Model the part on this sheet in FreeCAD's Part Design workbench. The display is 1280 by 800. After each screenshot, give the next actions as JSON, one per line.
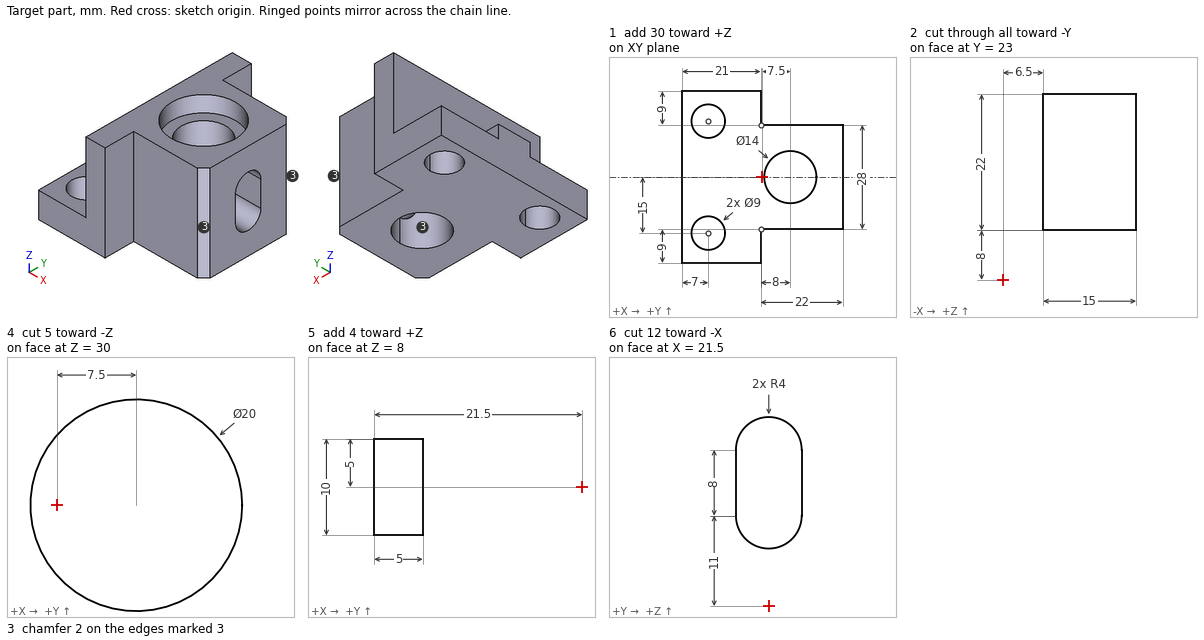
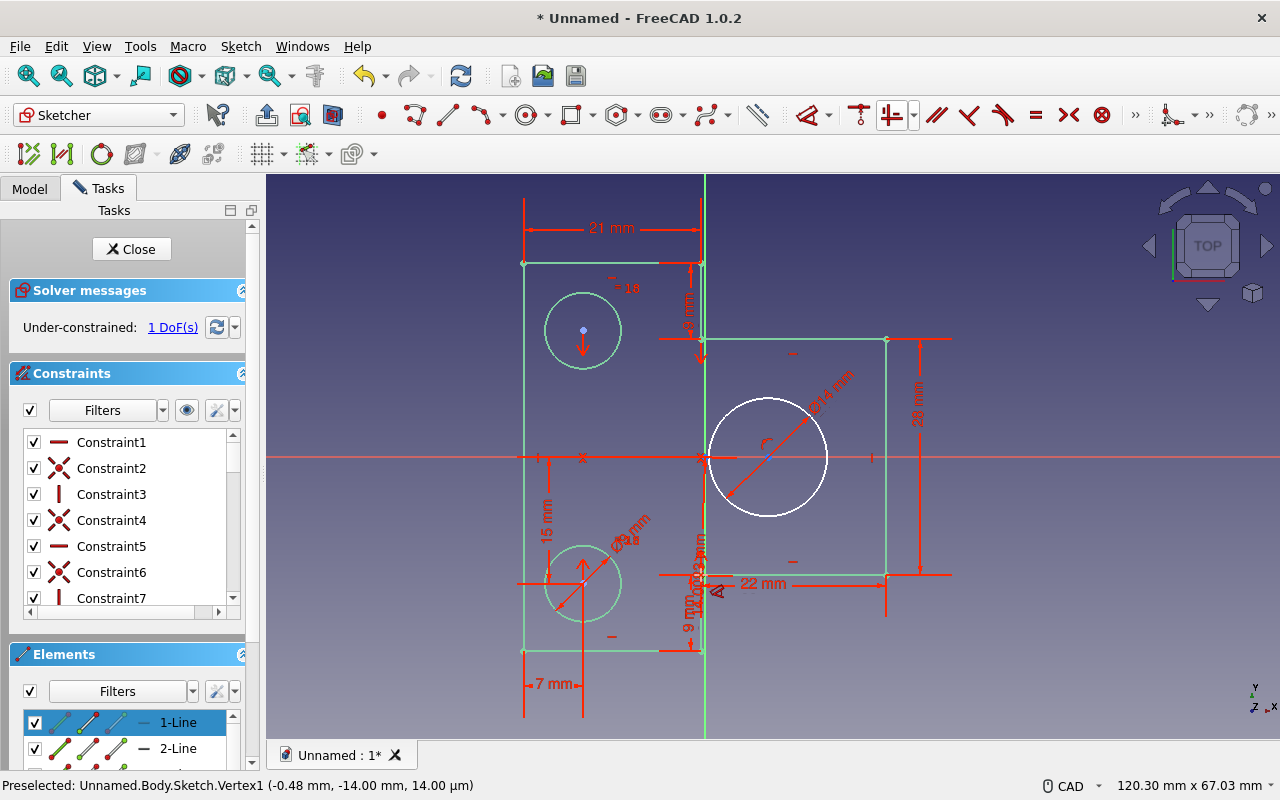
{"action": "left_click", "coordinate": [768, 457]}
{"action": "left_click", "coordinate": [750, 423]}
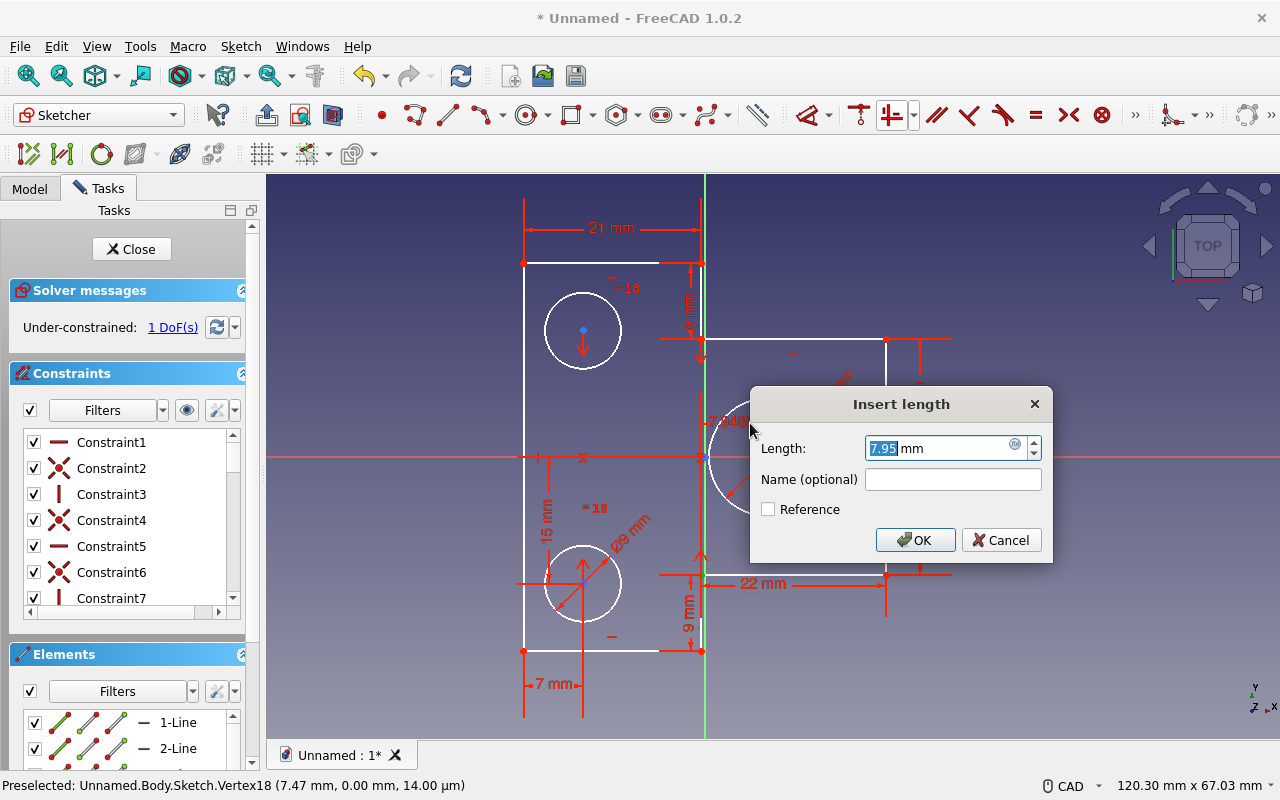
{"action": "type", "text": "8"}
{"action": "key", "text": "Return"}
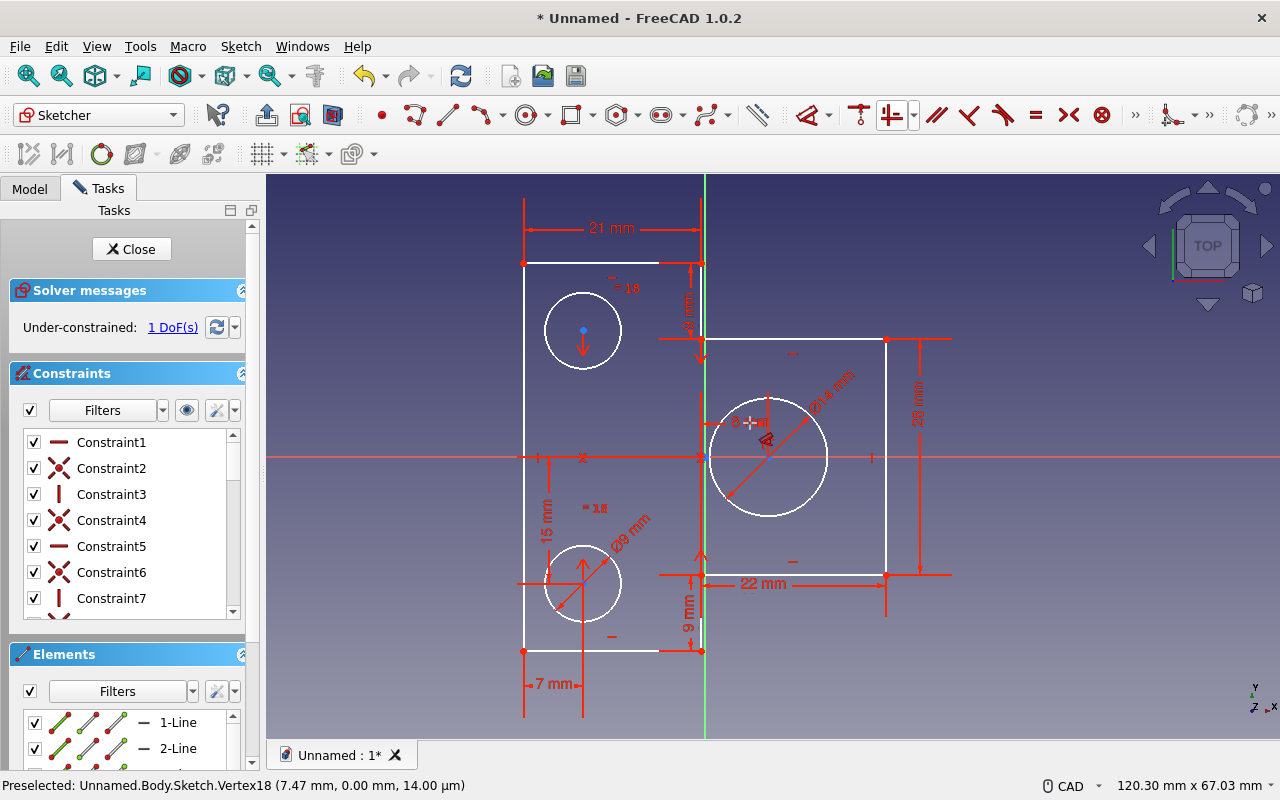
{"action": "left_click", "coordinate": [768, 457]}
{"action": "left_click", "coordinate": [751, 491]}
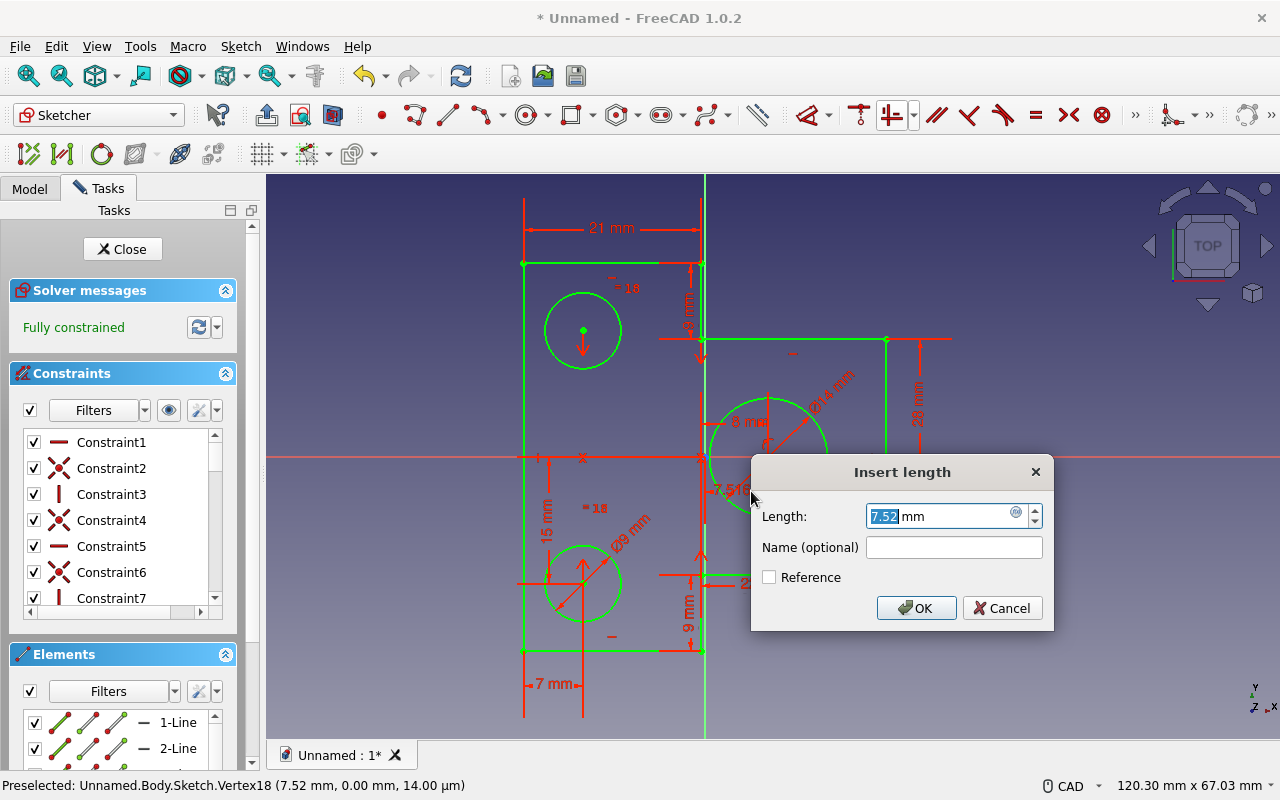
{"action": "type", "text": "7.5"}
{"action": "key", "text": "Return"}
{"action": "key", "text": "Escape"}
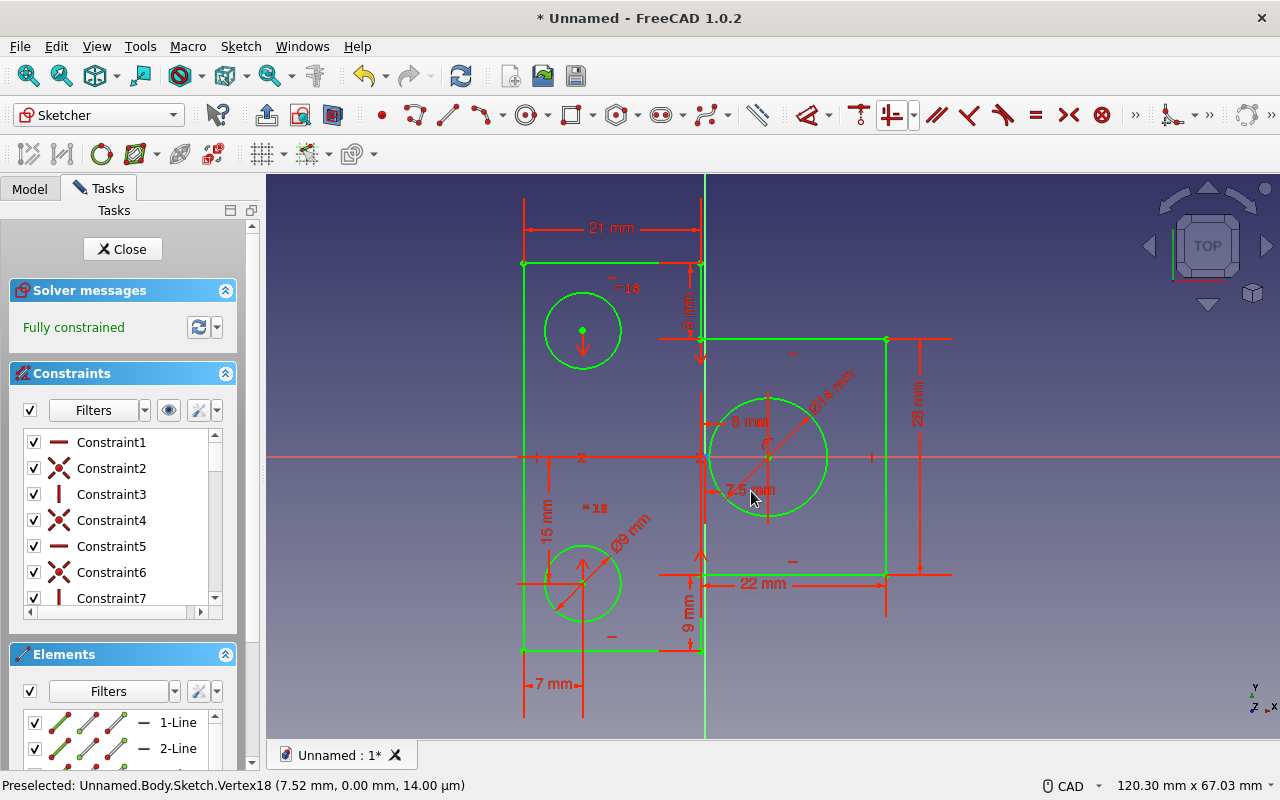
{"action": "left_click", "coordinate": [123, 249]}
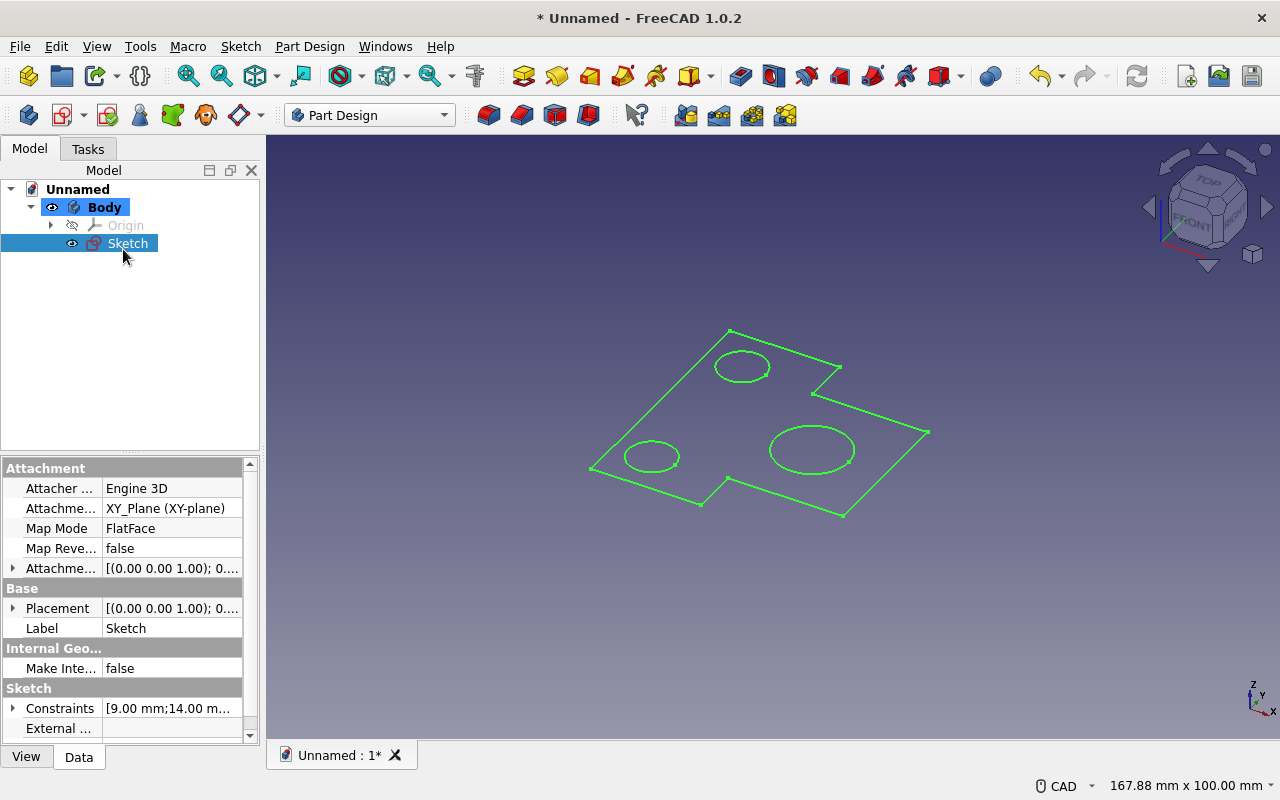
{"action": "left_click", "coordinate": [524, 76]}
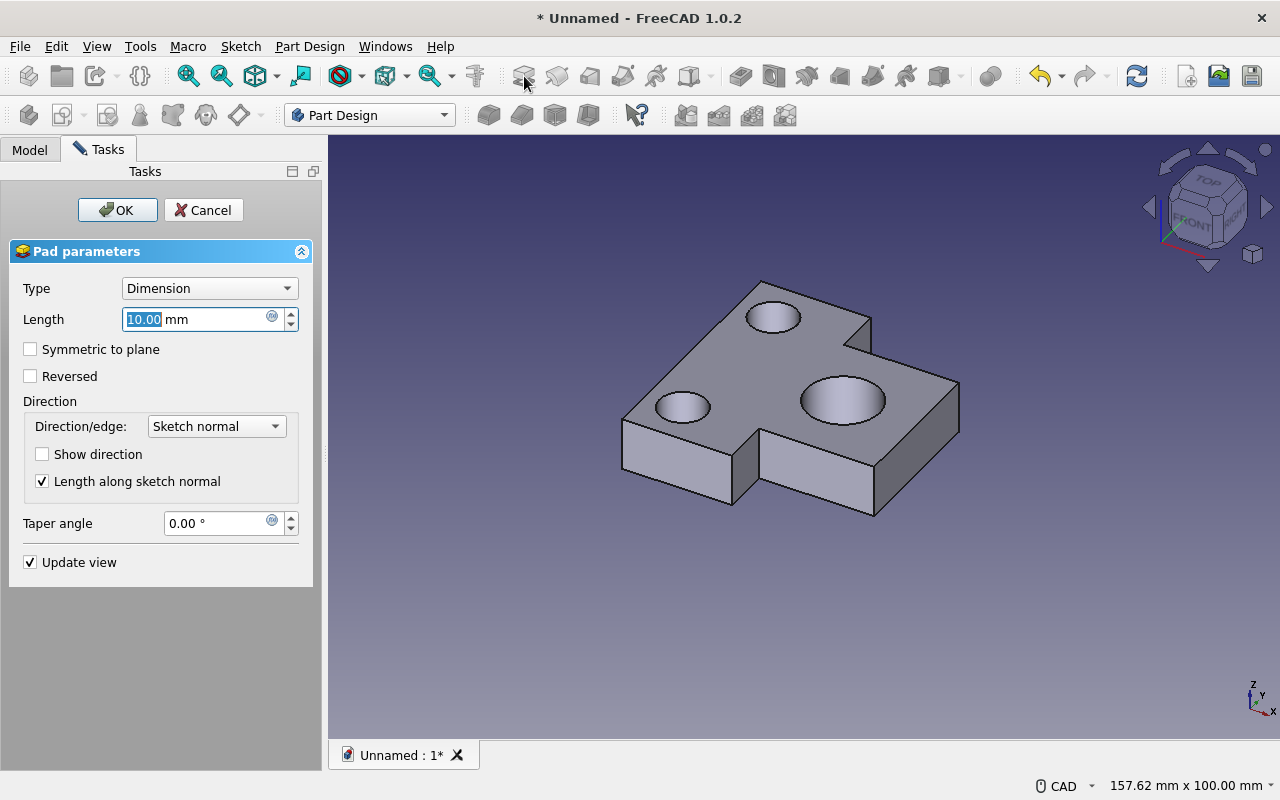
{"action": "type", "text": "30"}
{"action": "key", "text": "Tab"}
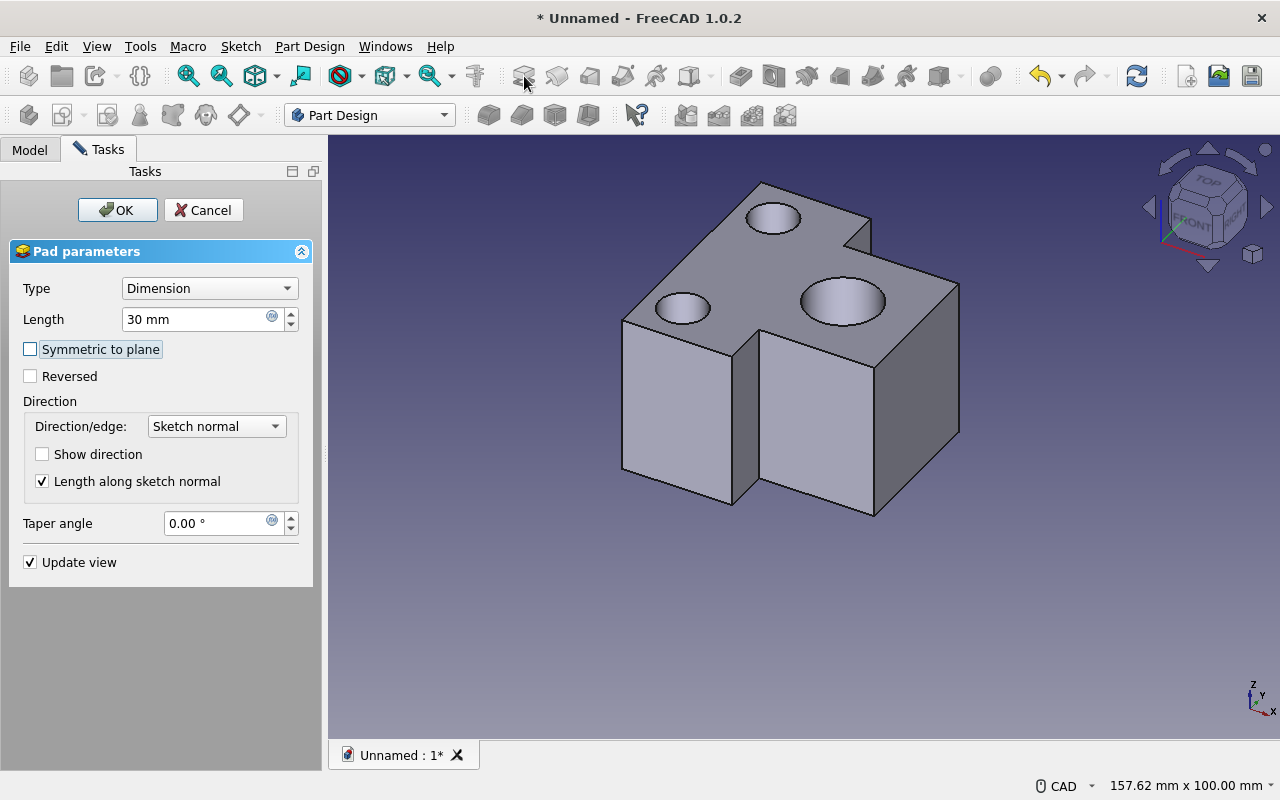
{"action": "left_click", "coordinate": [118, 210]}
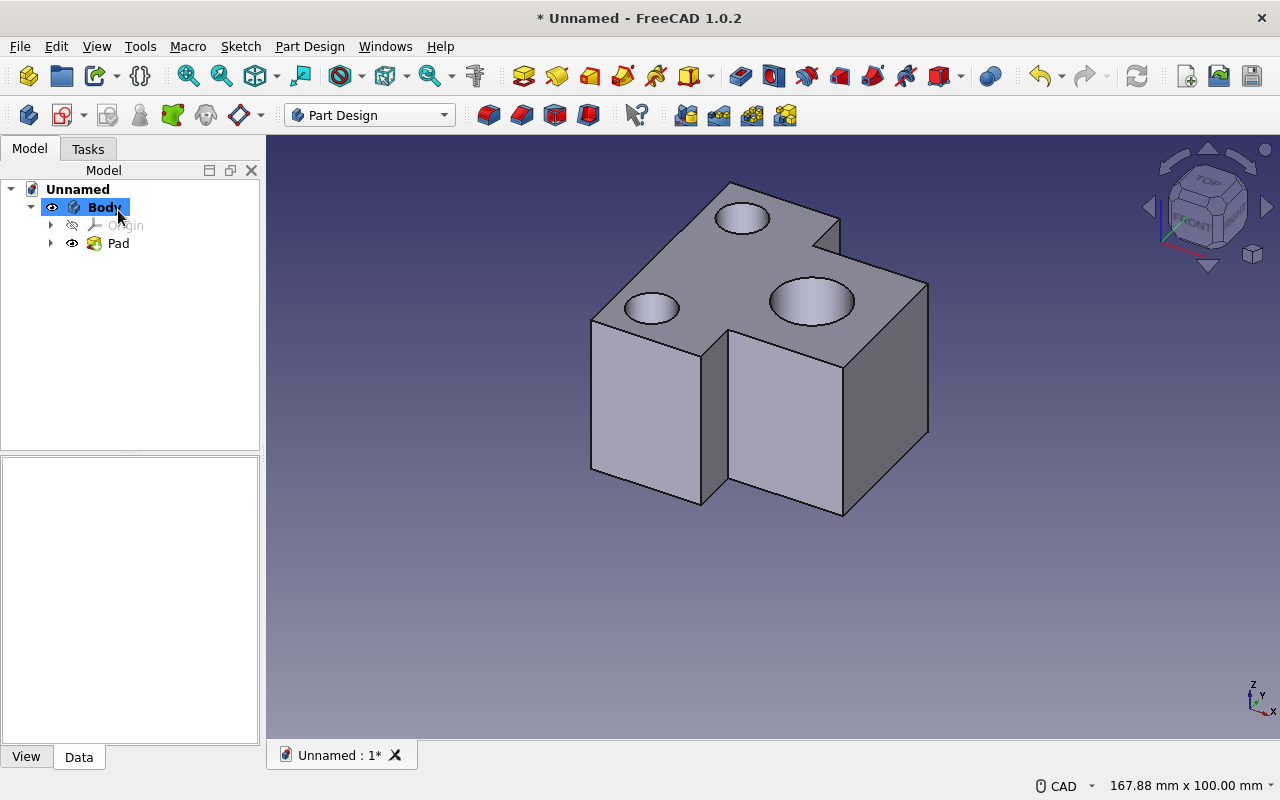
{"action": "key", "text": "4"}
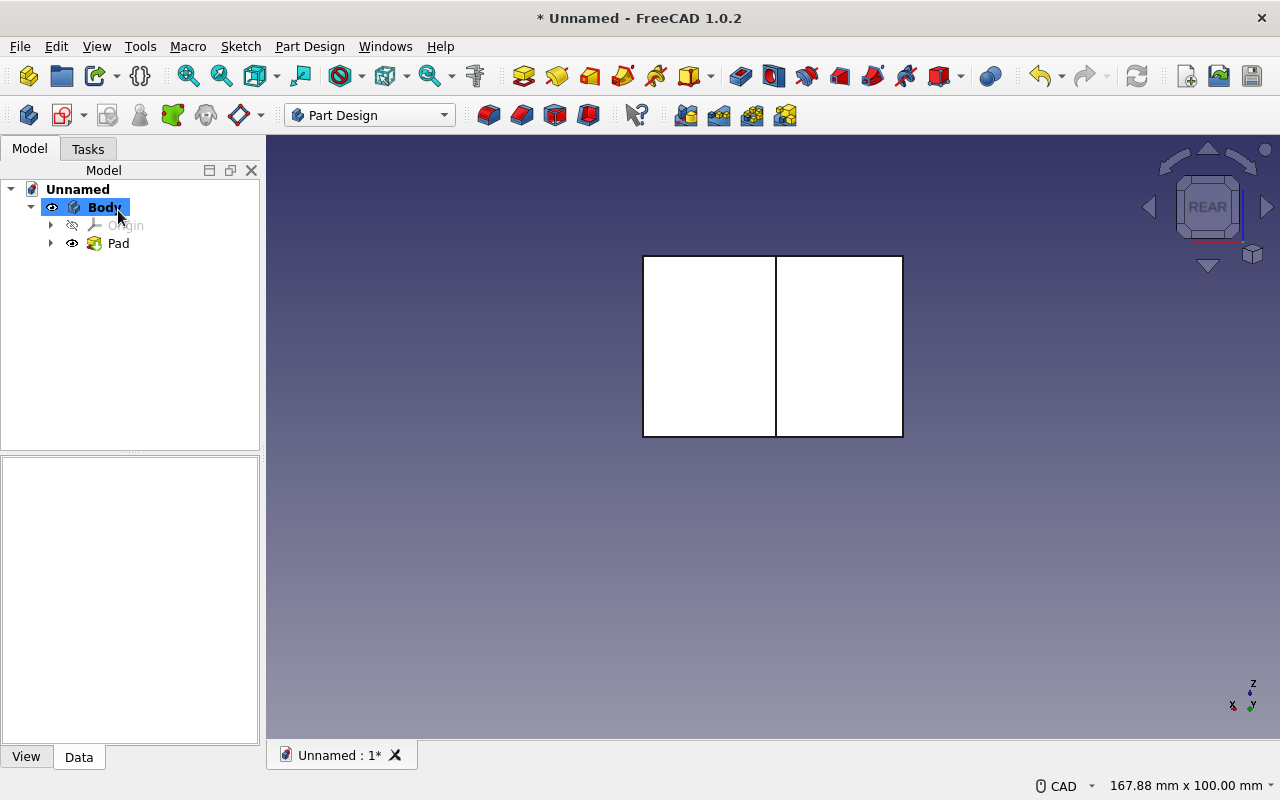
{"action": "left_click", "coordinate": [189, 76]}